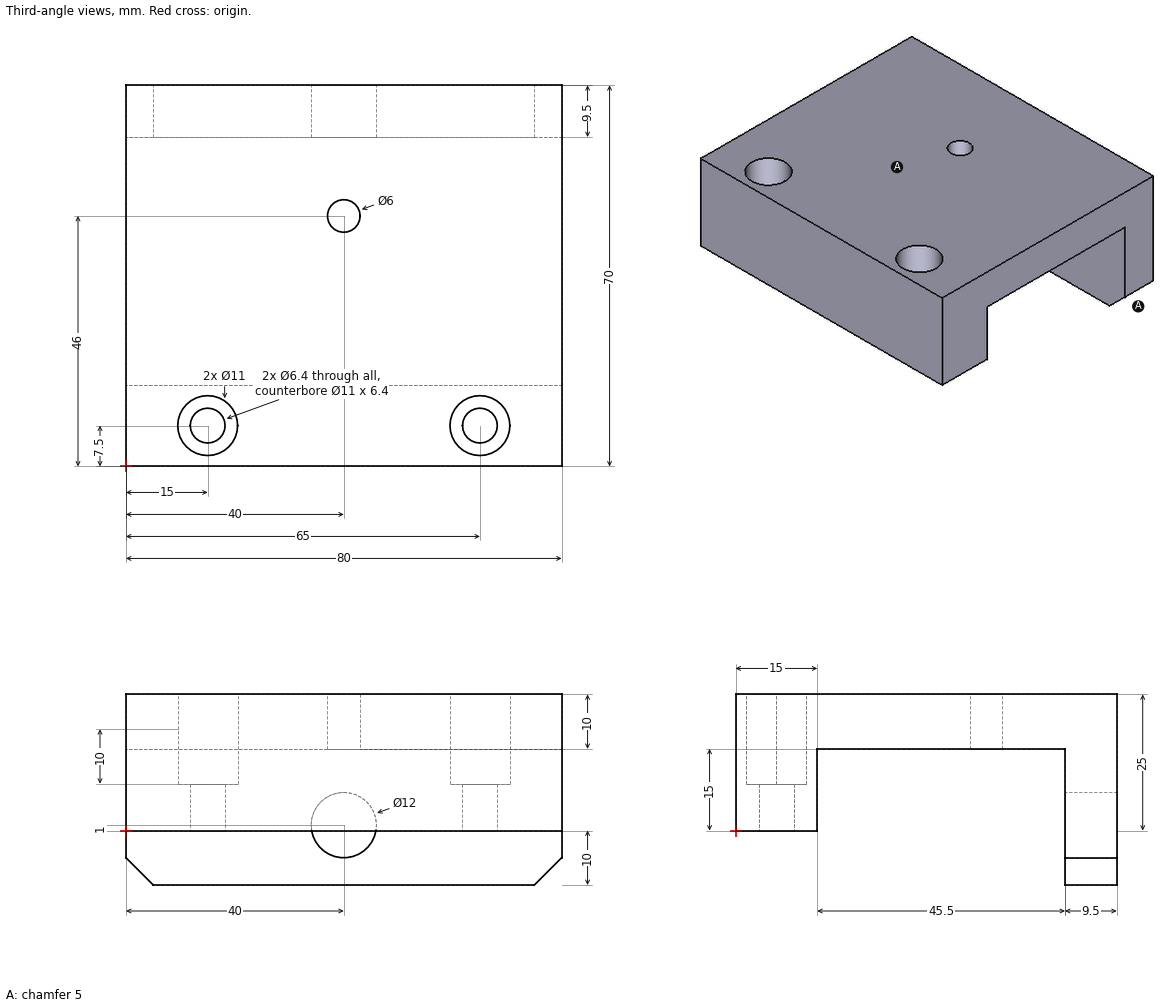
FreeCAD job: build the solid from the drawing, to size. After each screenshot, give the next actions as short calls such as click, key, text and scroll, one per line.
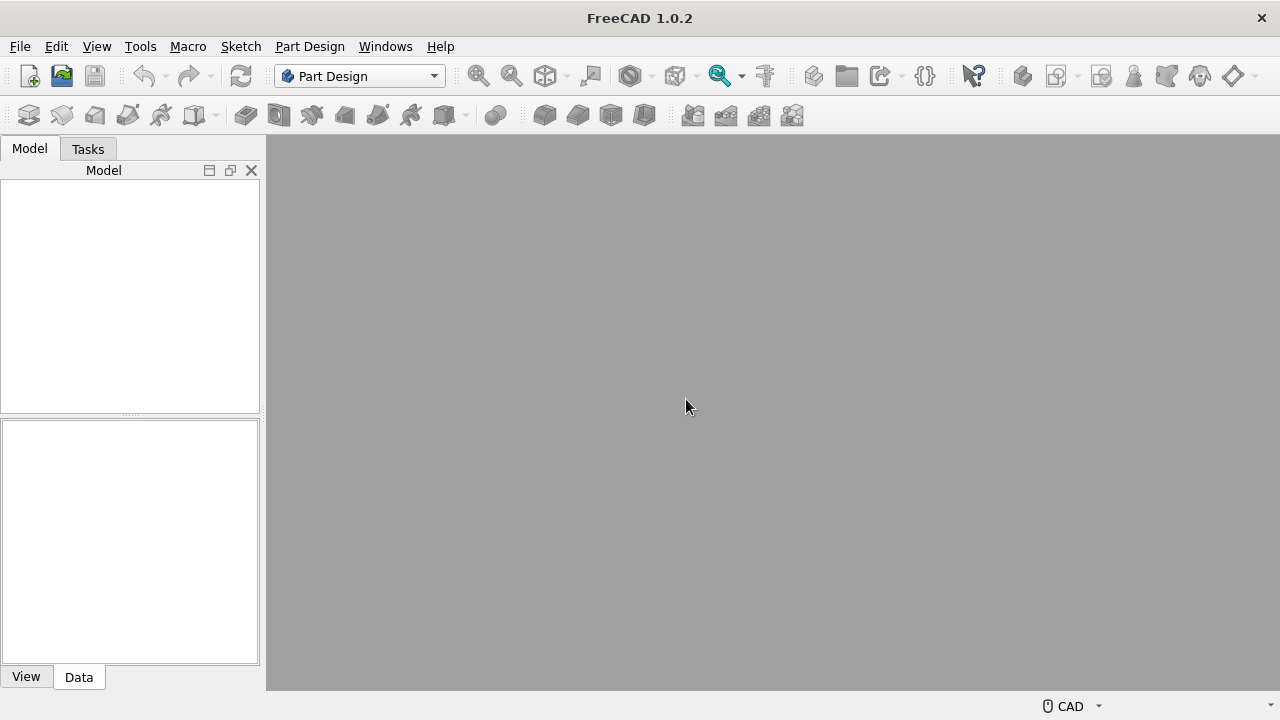
click(29, 76)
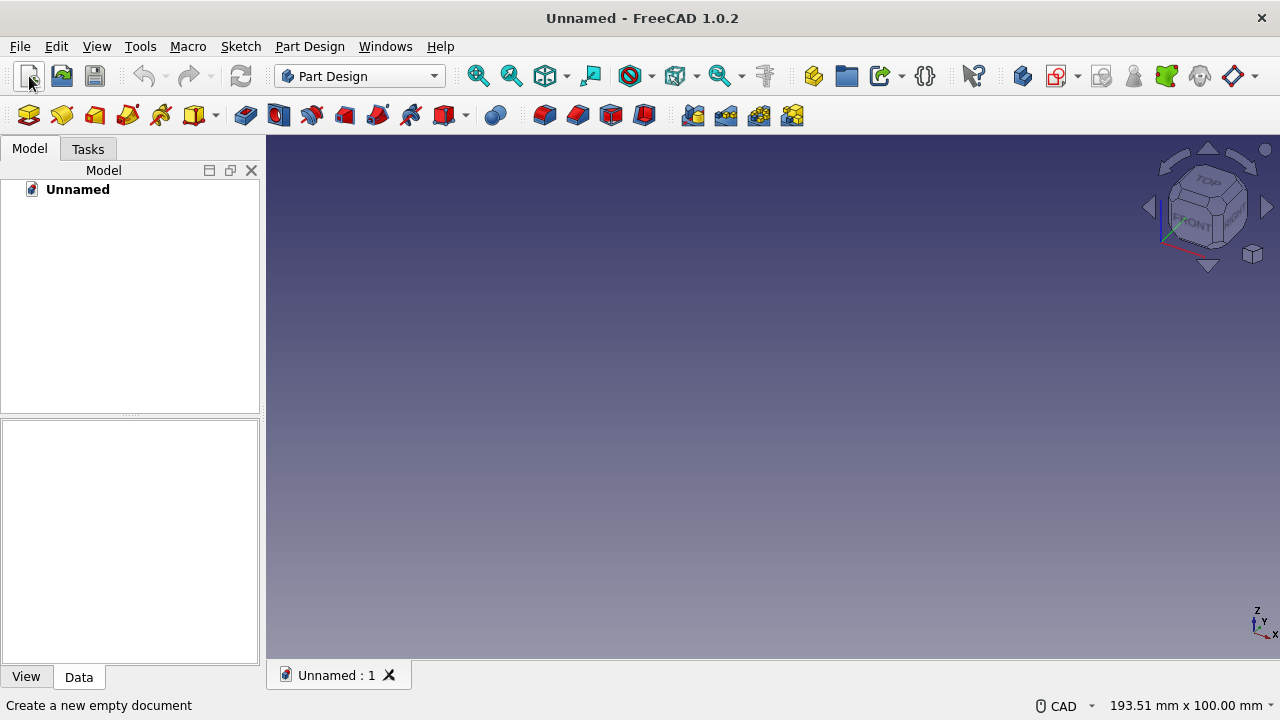
click(1056, 76)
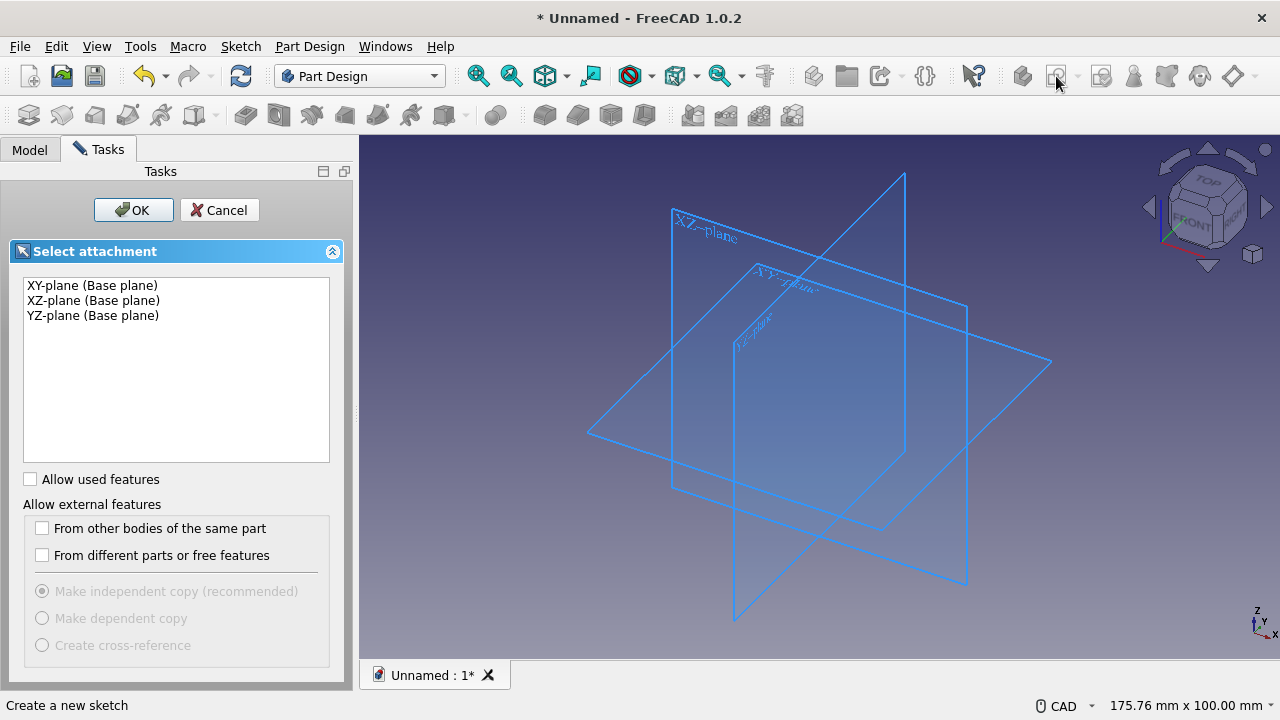
click(84, 286)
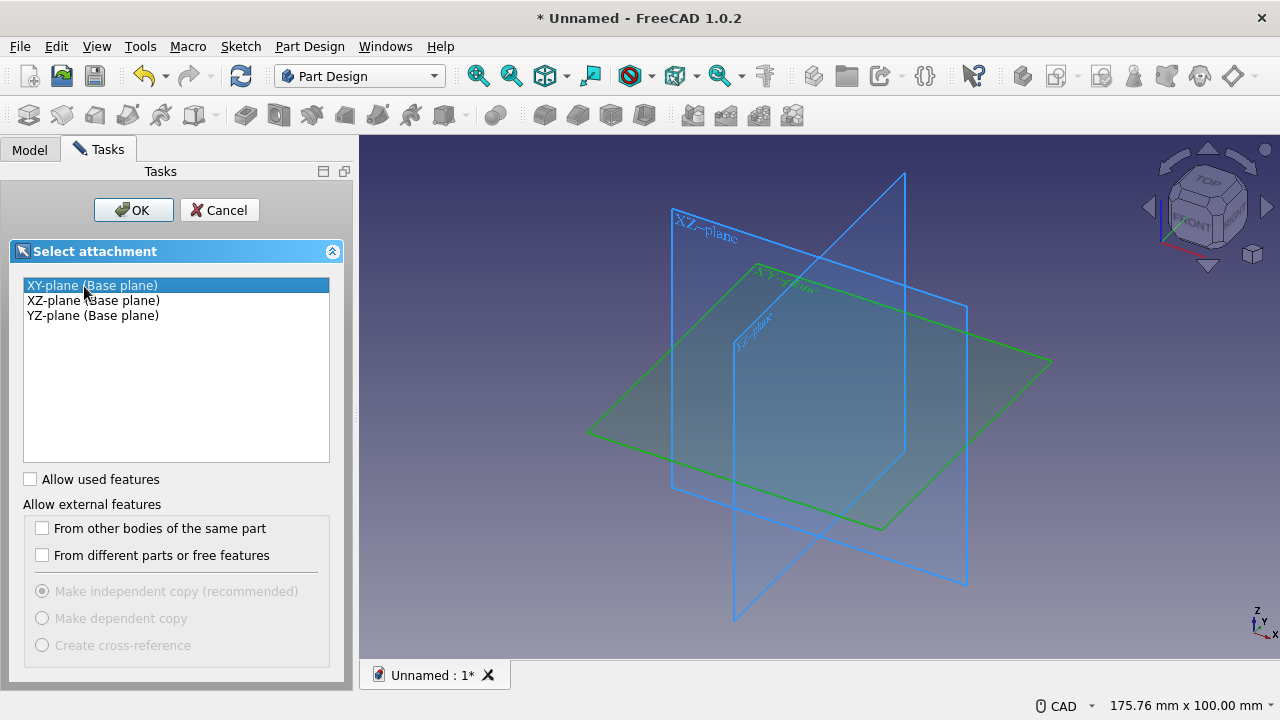
click(134, 210)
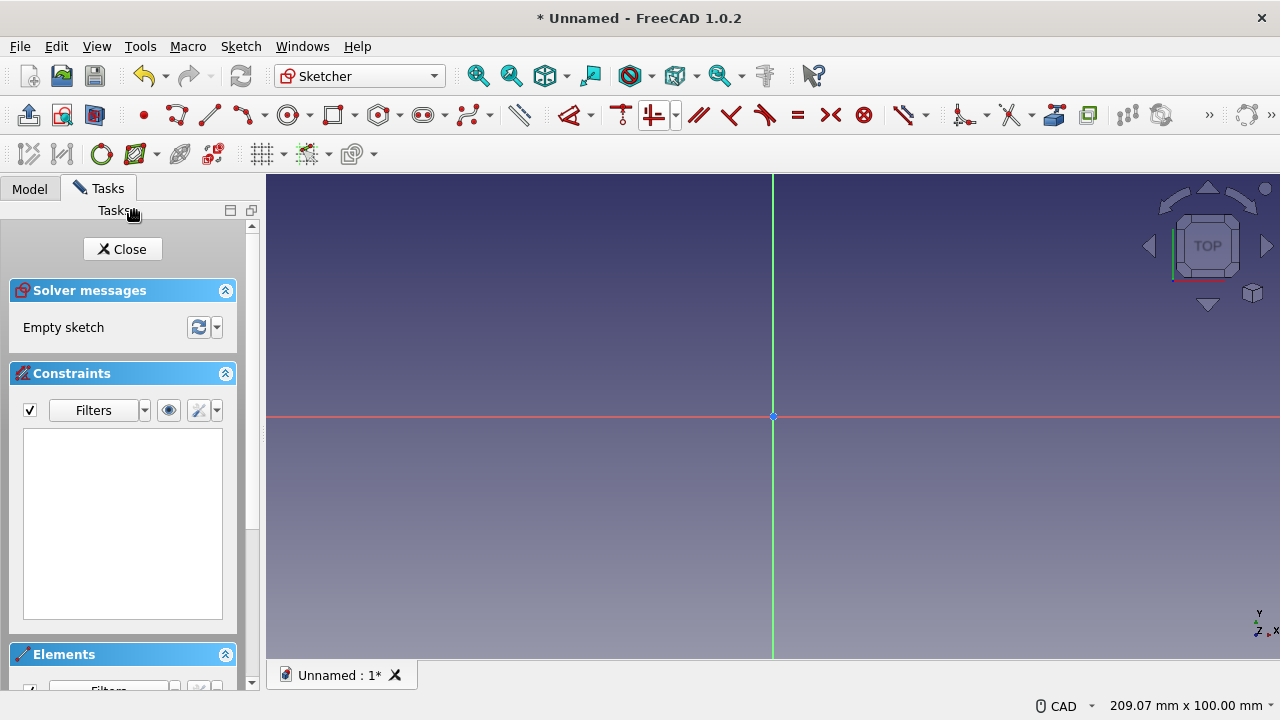
scroll(294, 631, down, 2)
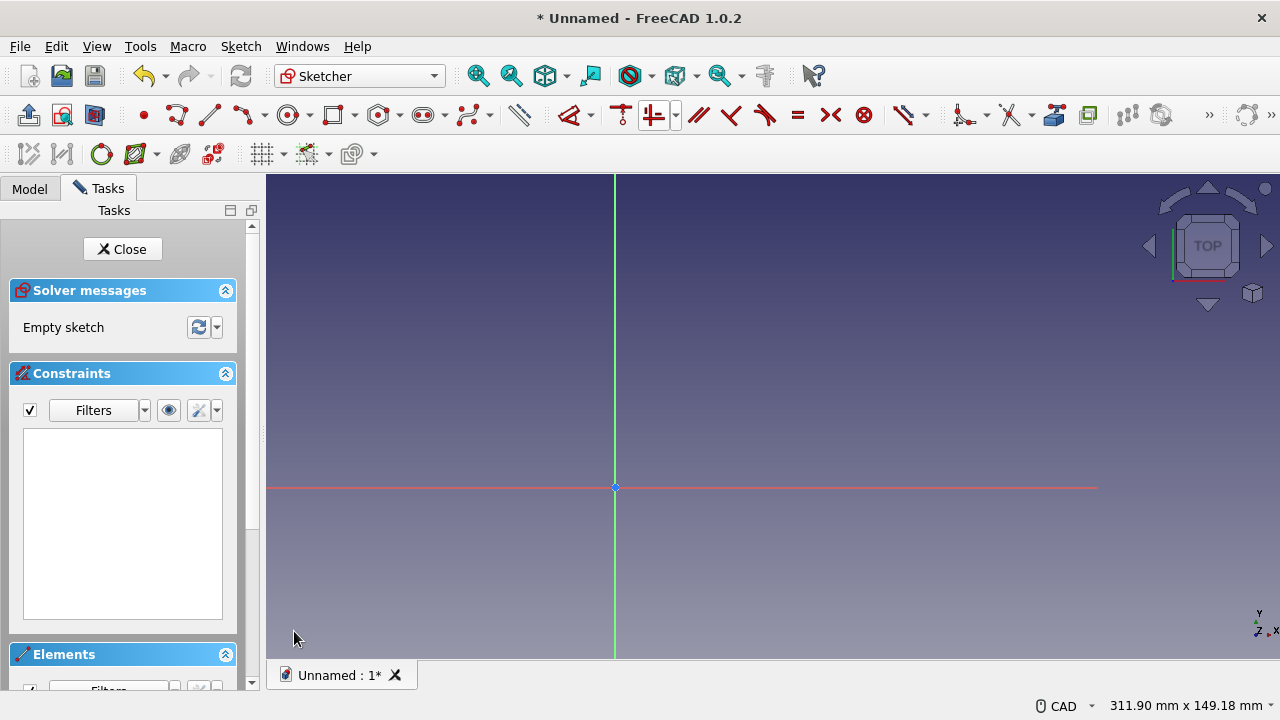
click(332, 116)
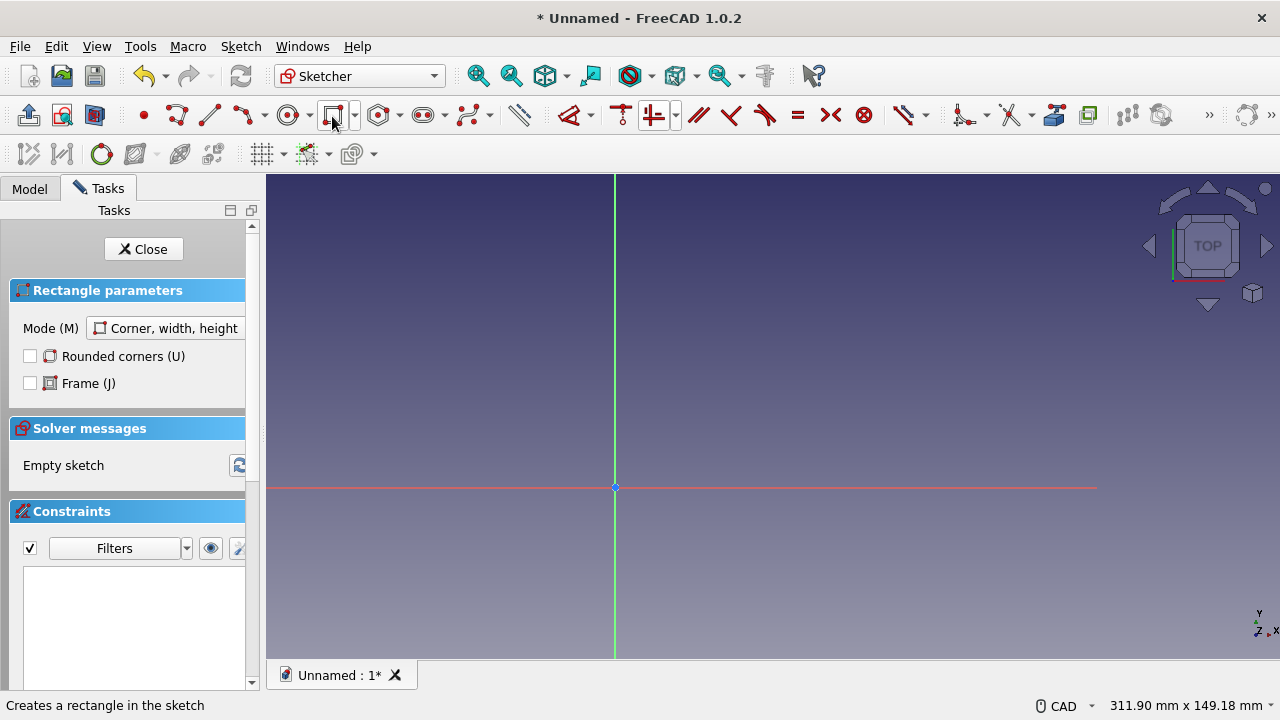
click(615, 488)
move(875, 260)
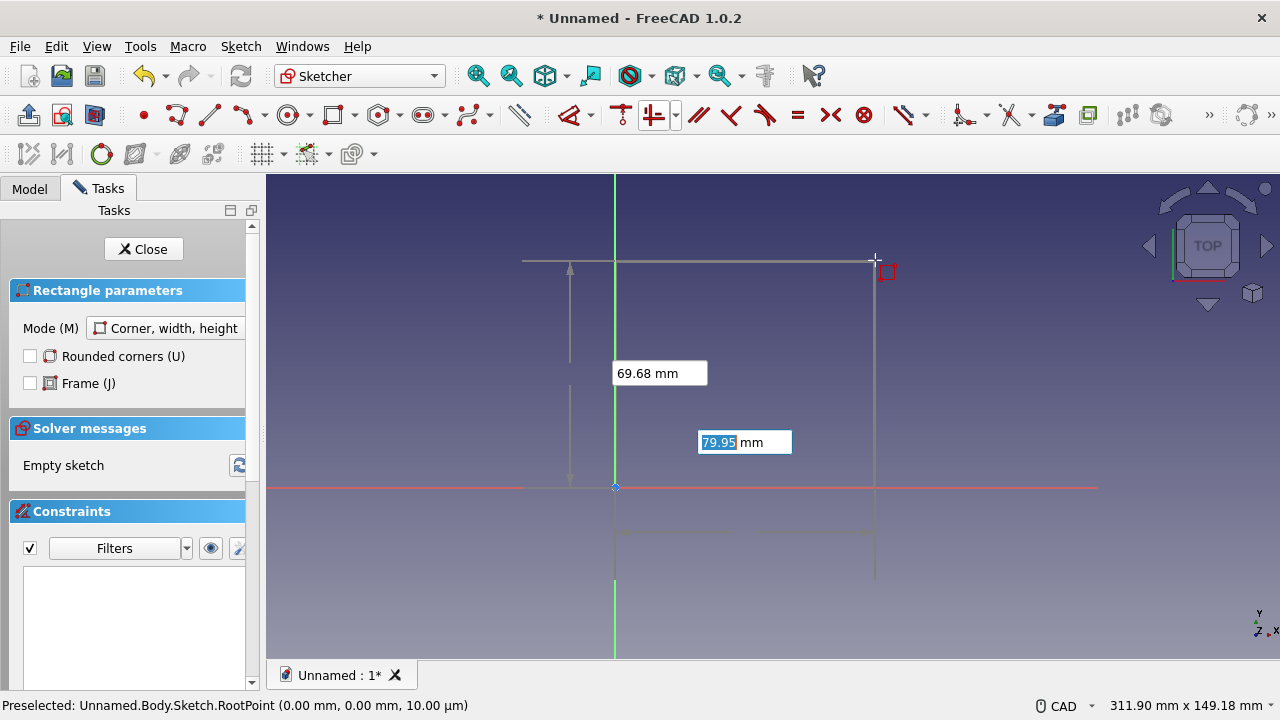
text(80)
key(Tab)
text(70)
key(Return)
key(Escape)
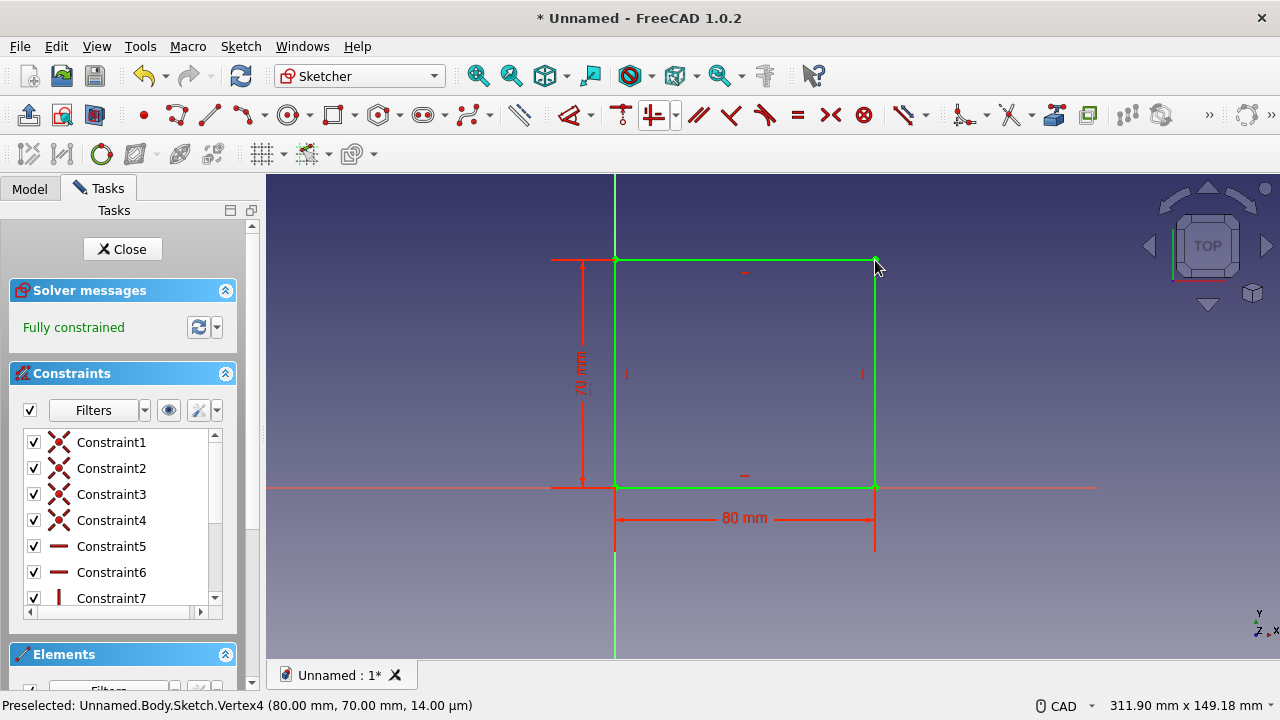
click(123, 249)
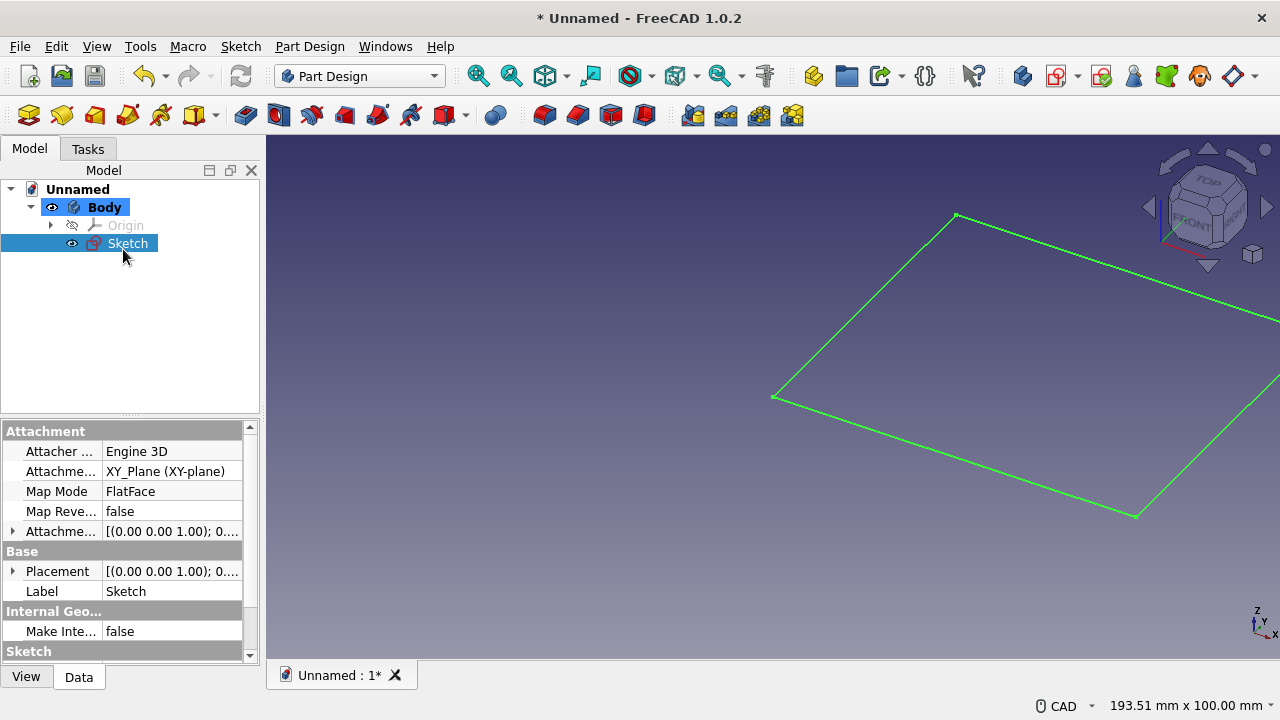
click(29, 116)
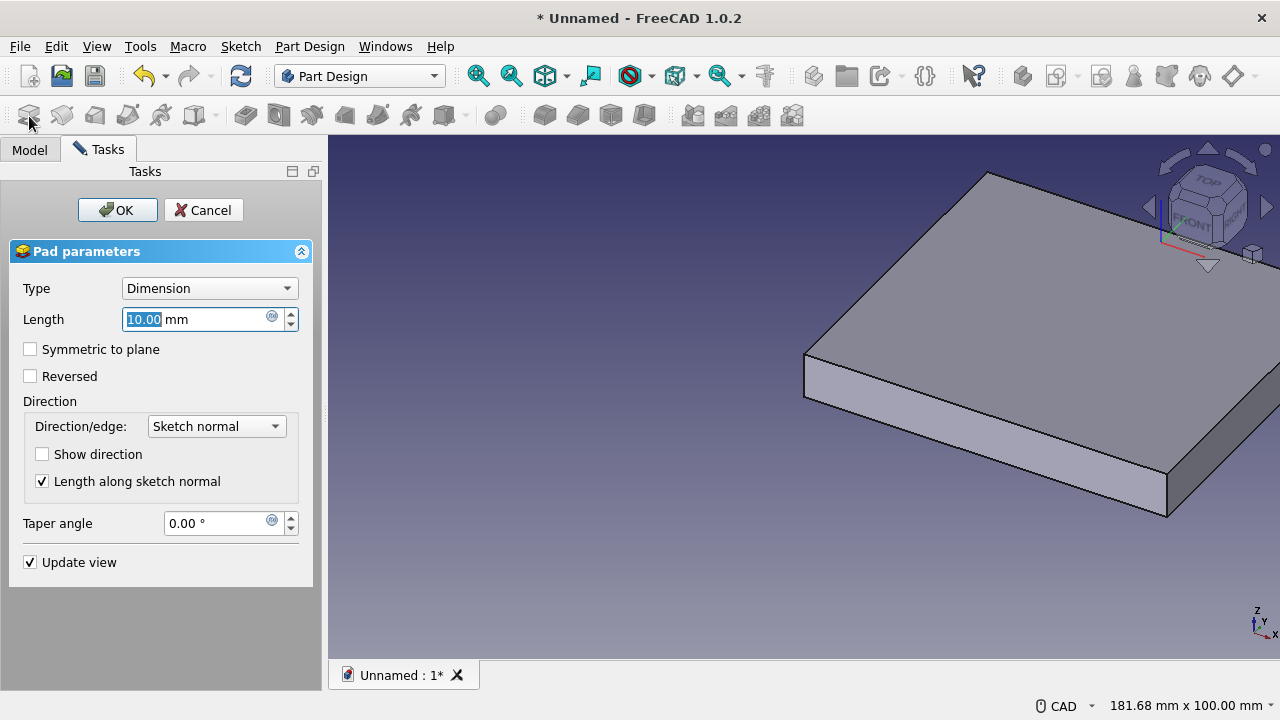
text(25)
key(Tab)